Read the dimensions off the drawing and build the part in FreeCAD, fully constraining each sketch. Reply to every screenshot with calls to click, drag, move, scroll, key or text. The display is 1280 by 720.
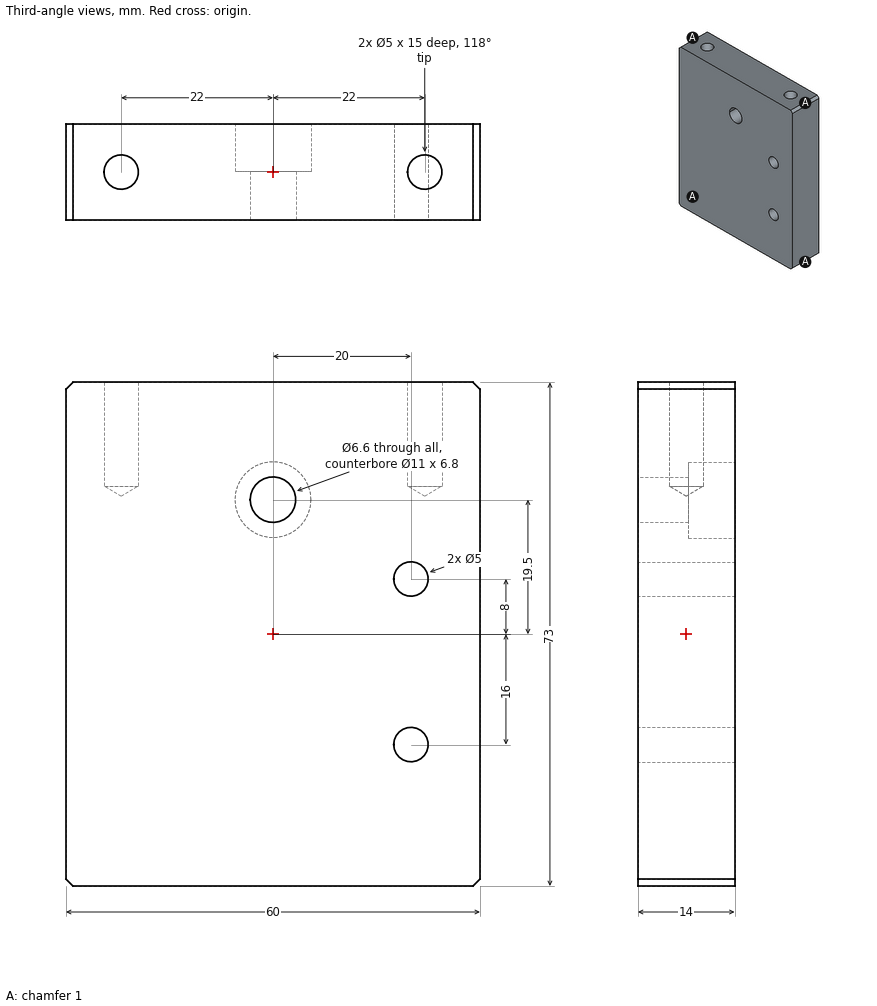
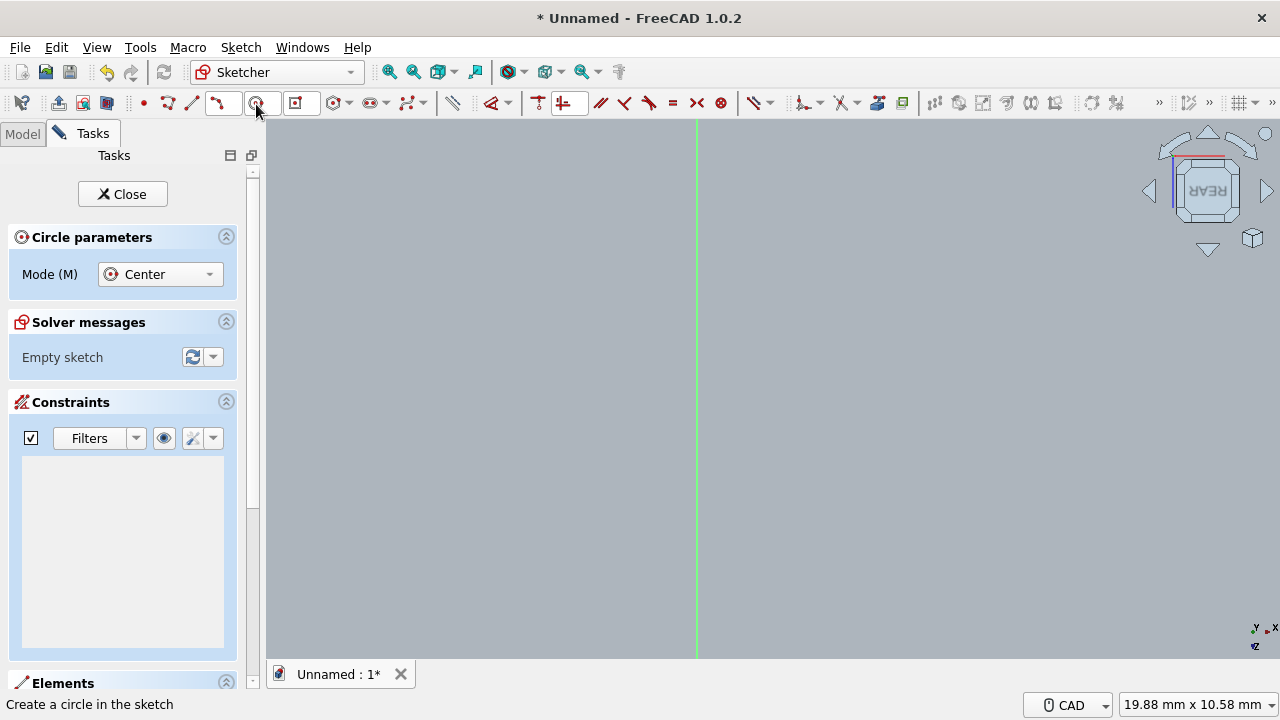
click(697, 383)
click(816, 264)
key(Escape)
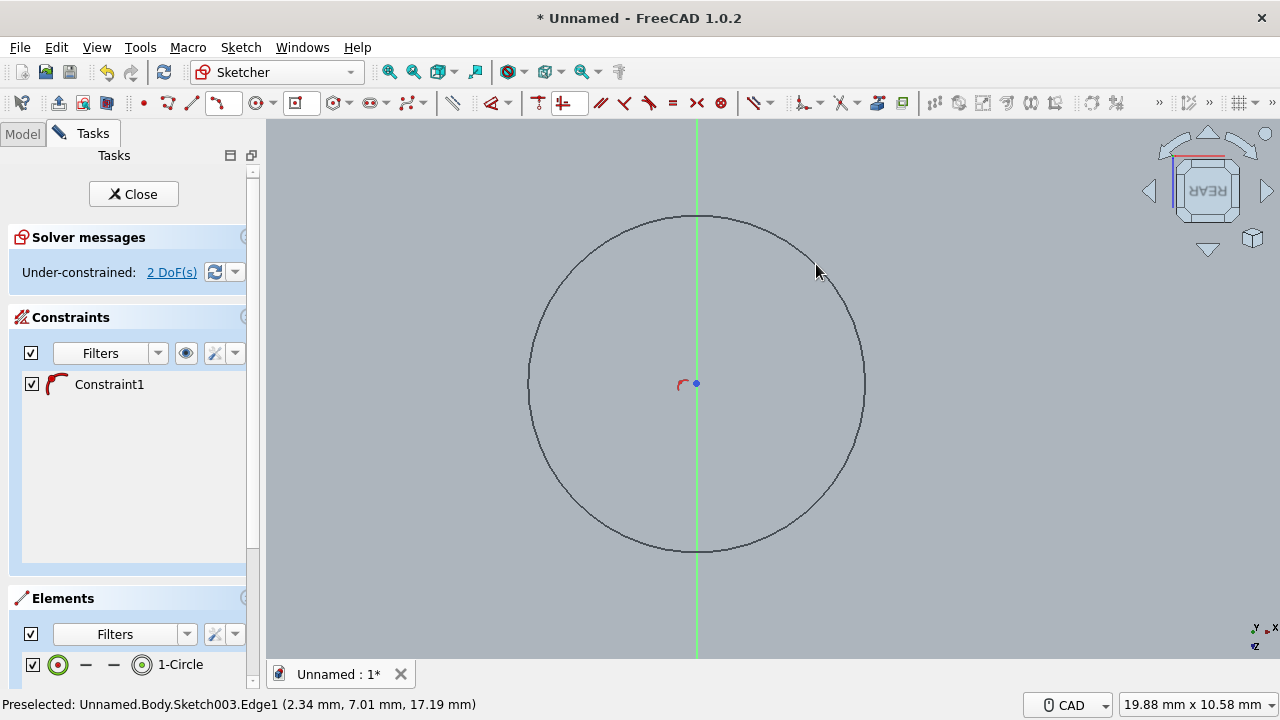
click(492, 104)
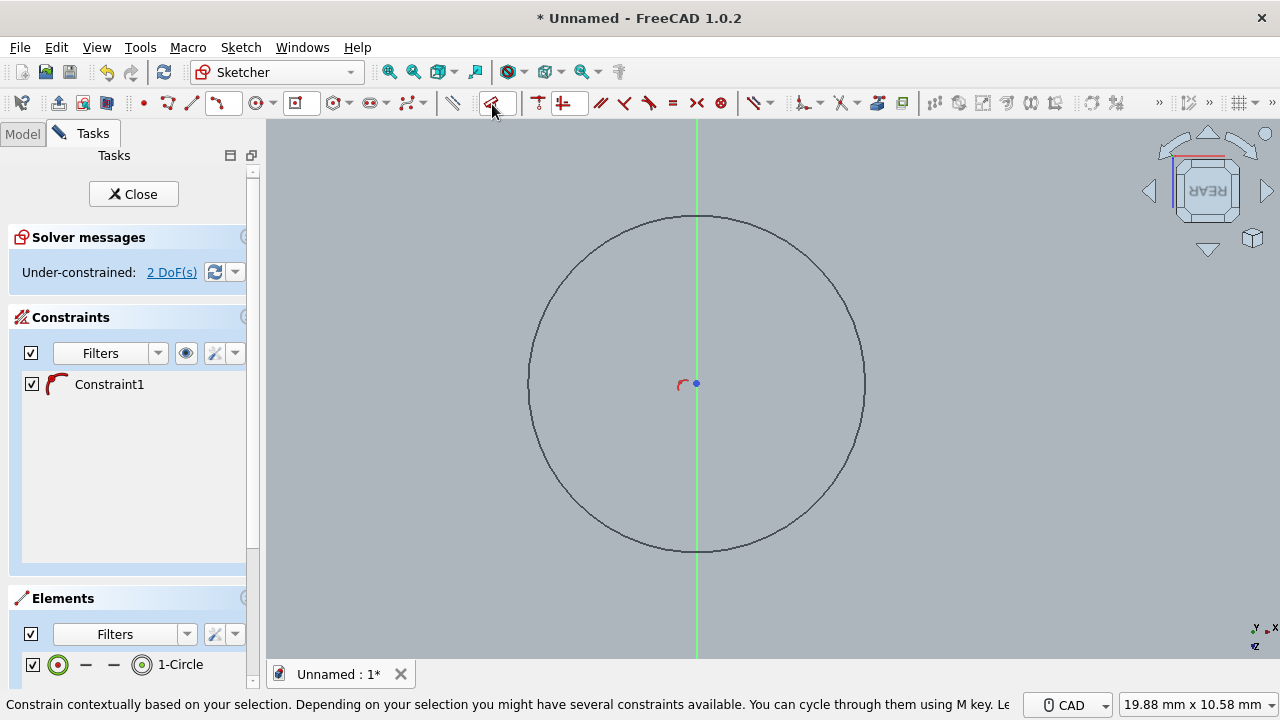
click(815, 264)
click(837, 241)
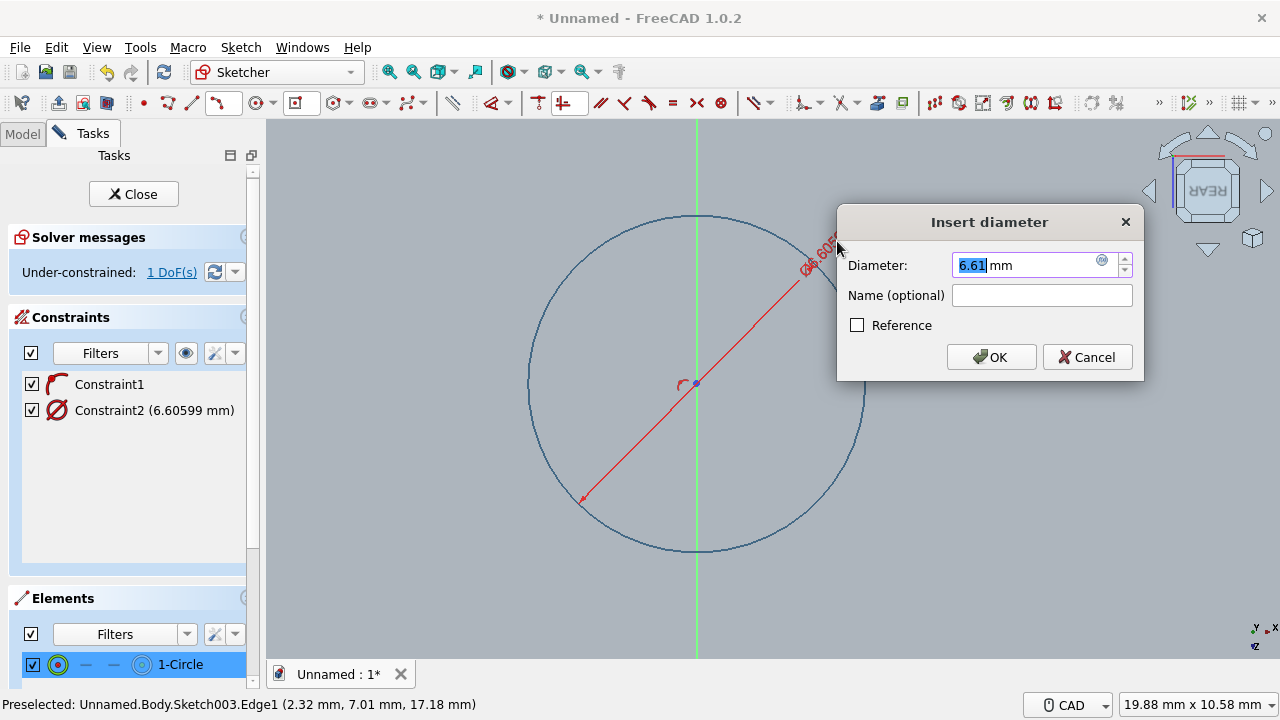
text(6.6)
key(Return)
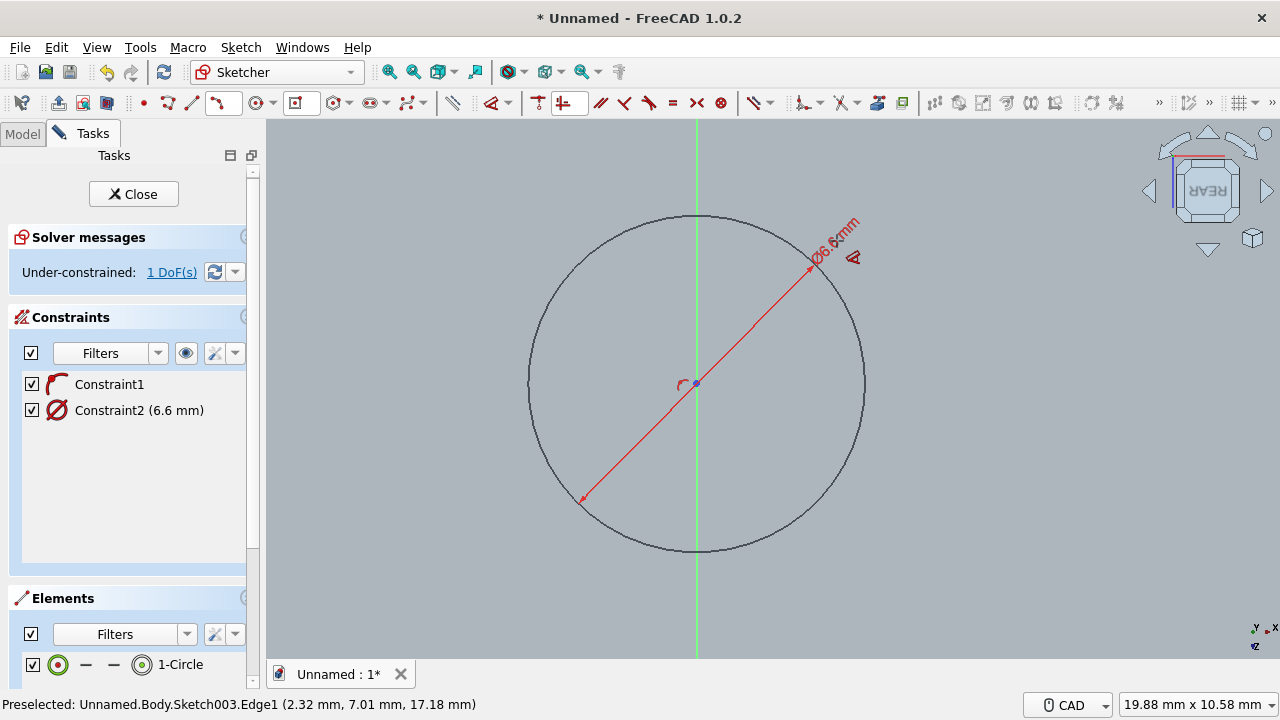
click(697, 384)
click(731, 265)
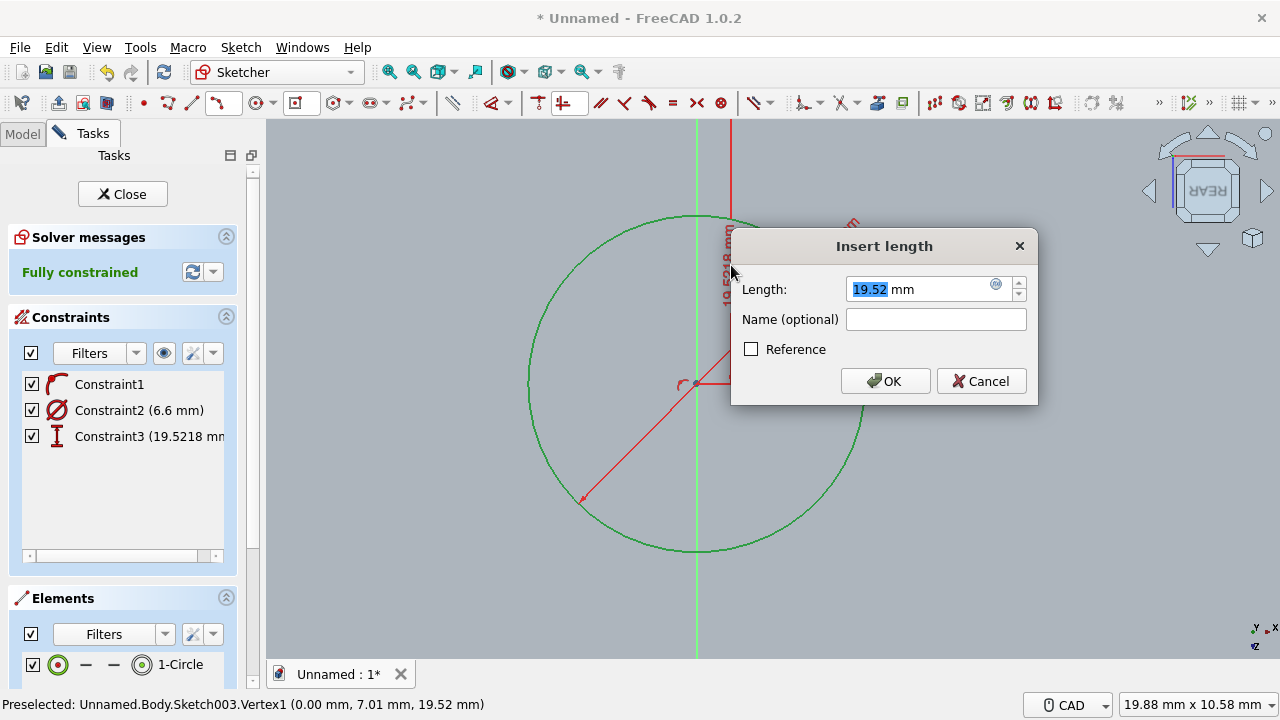
text(19.5)
key(Return)
key(Escape)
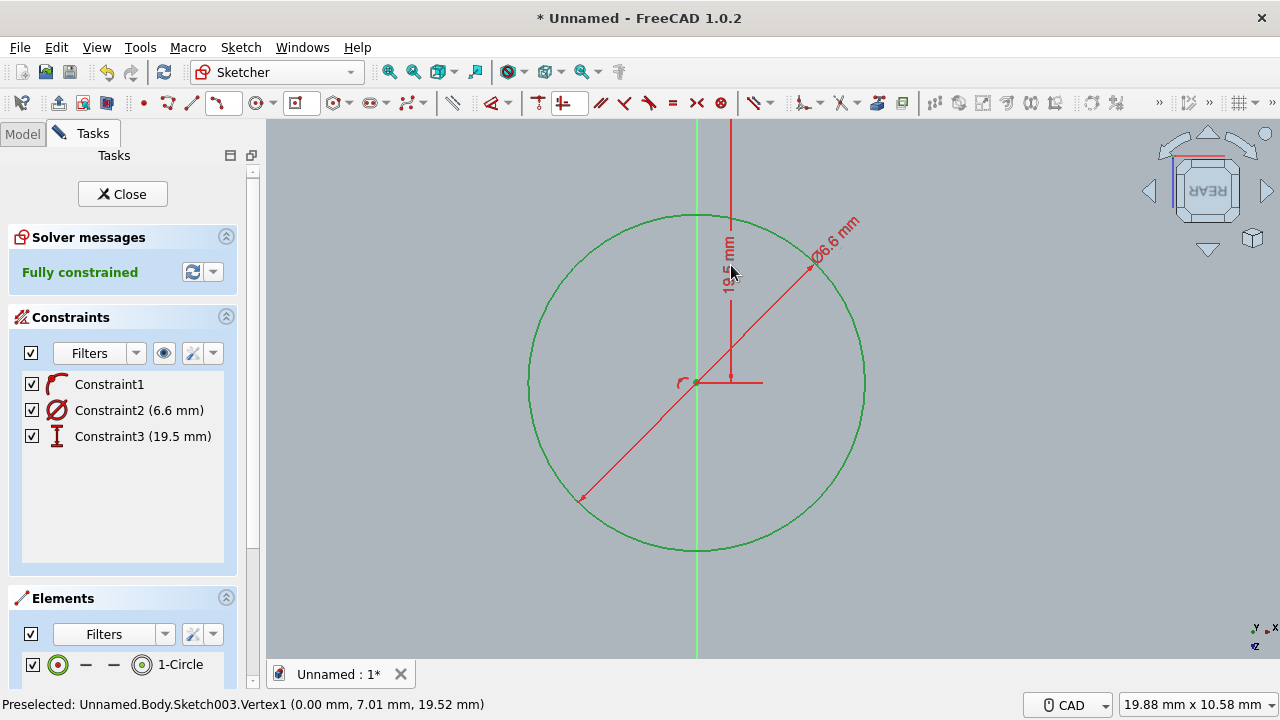
click(123, 194)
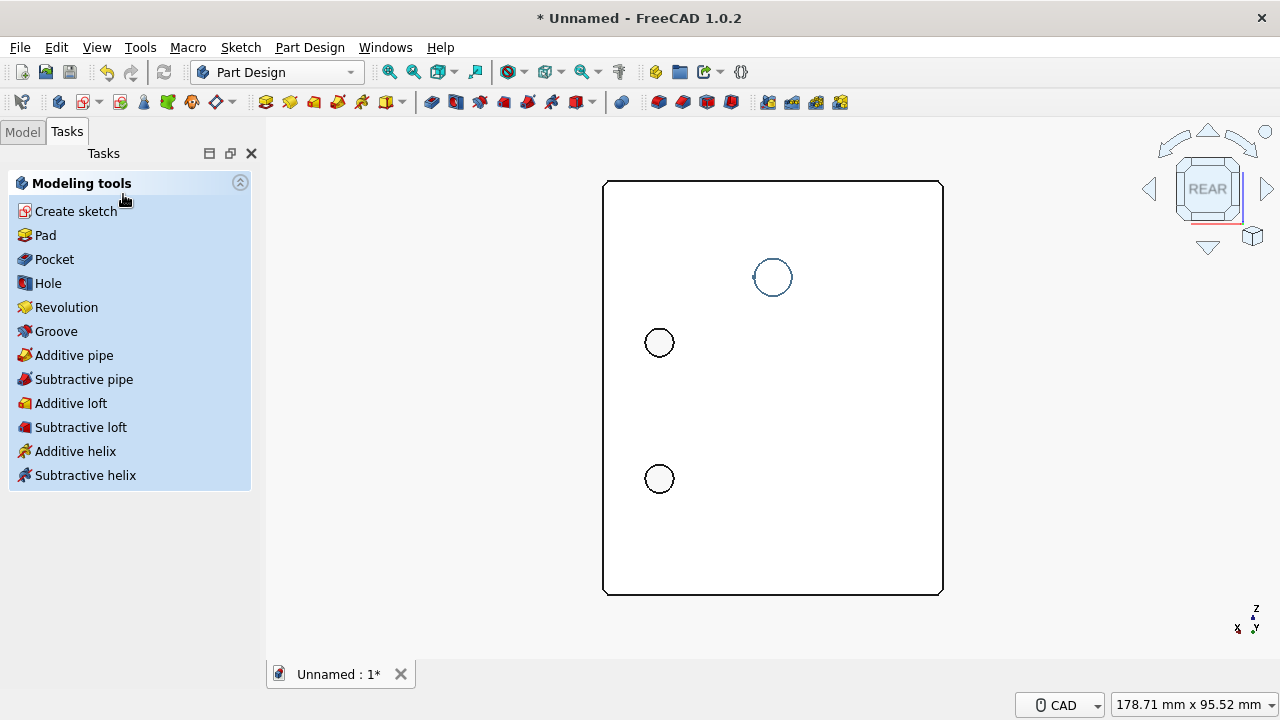
click(456, 102)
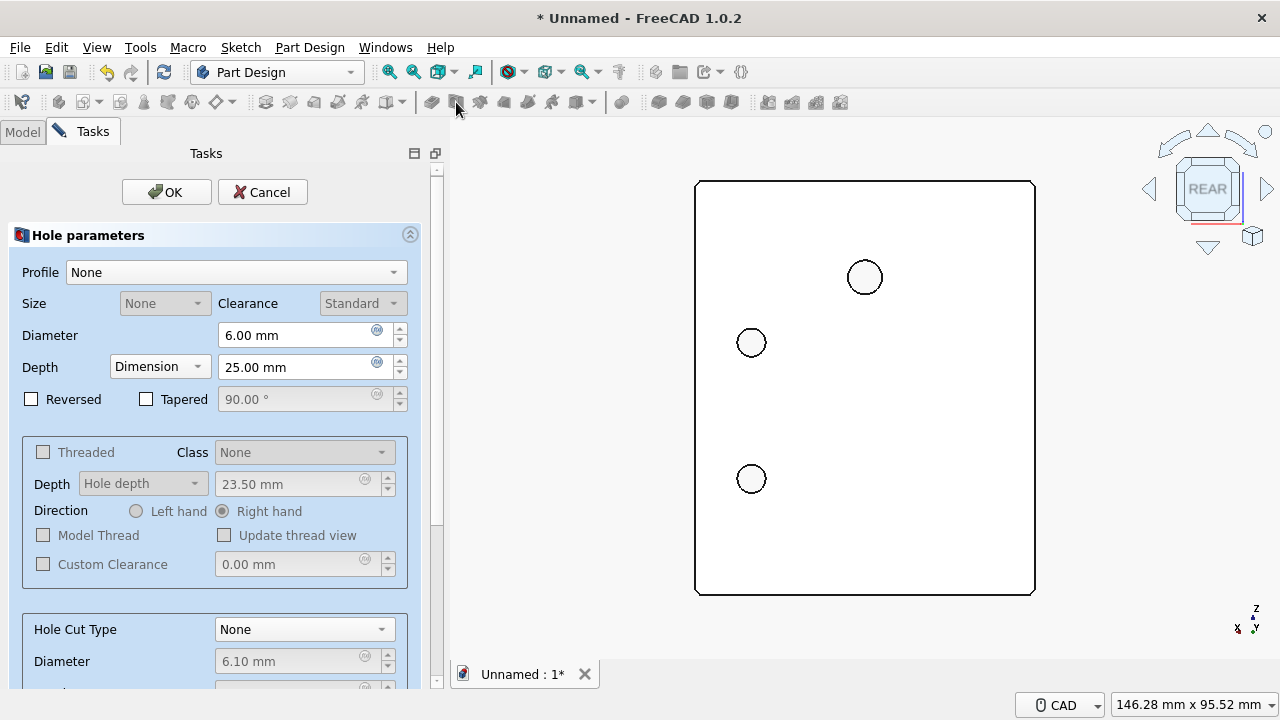
triple_click(305, 335)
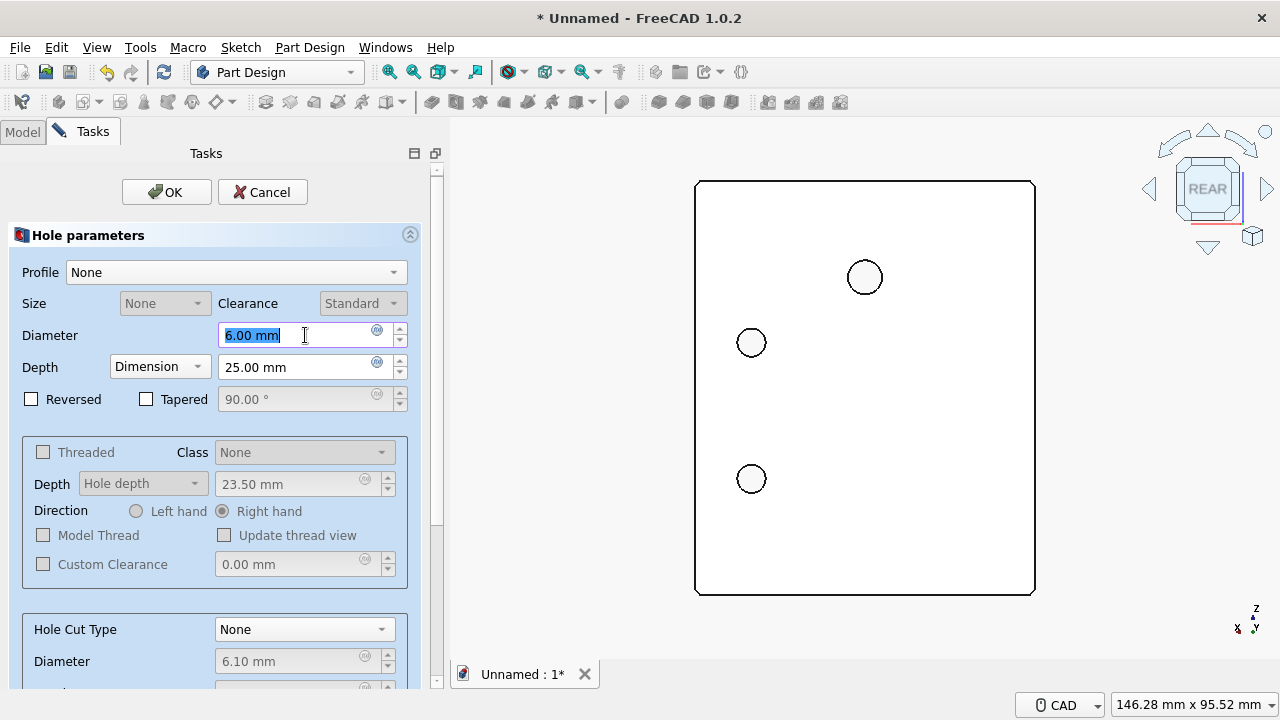
text(6.6)
key(Tab)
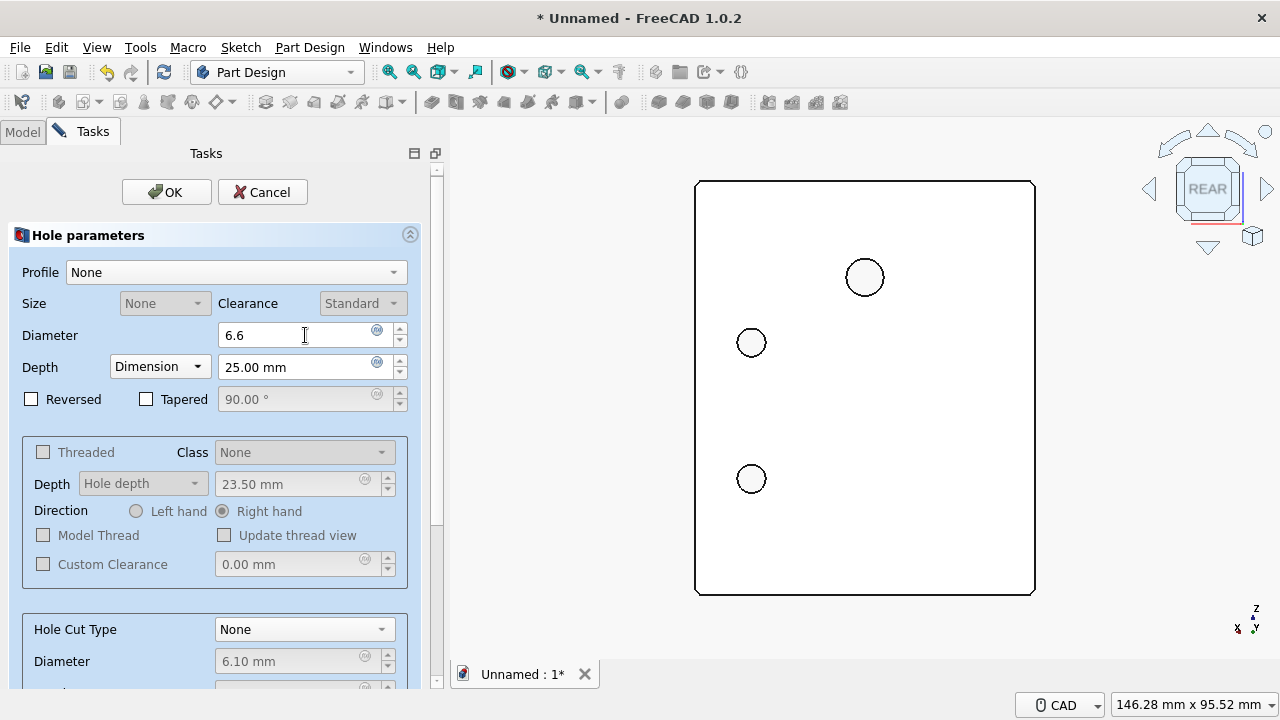
click(161, 366)